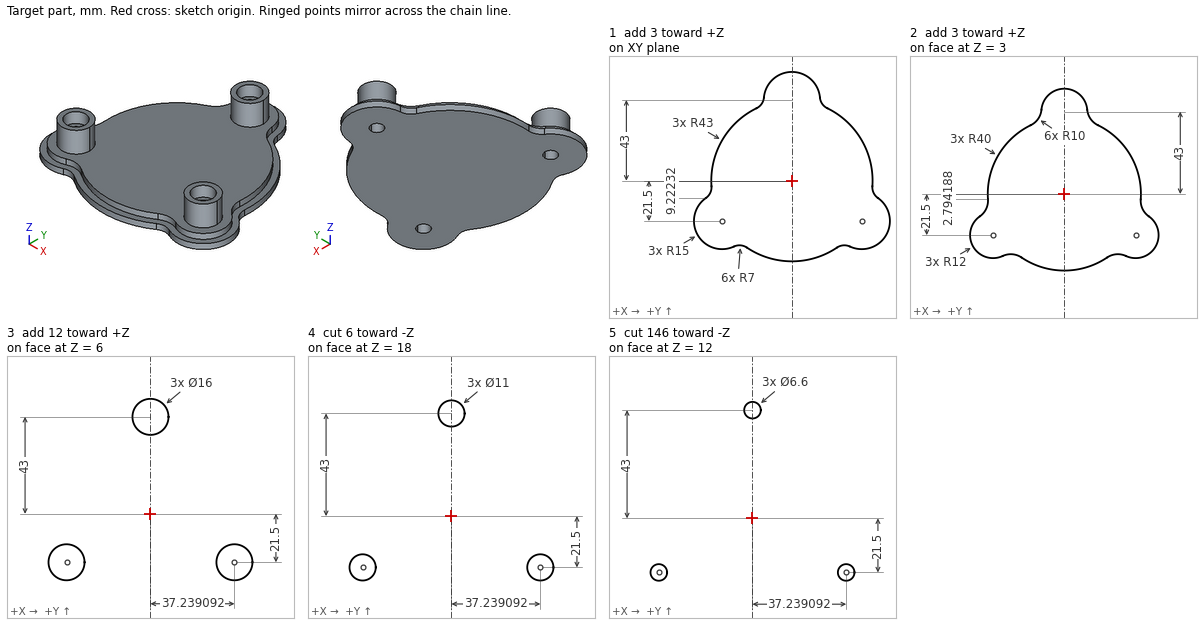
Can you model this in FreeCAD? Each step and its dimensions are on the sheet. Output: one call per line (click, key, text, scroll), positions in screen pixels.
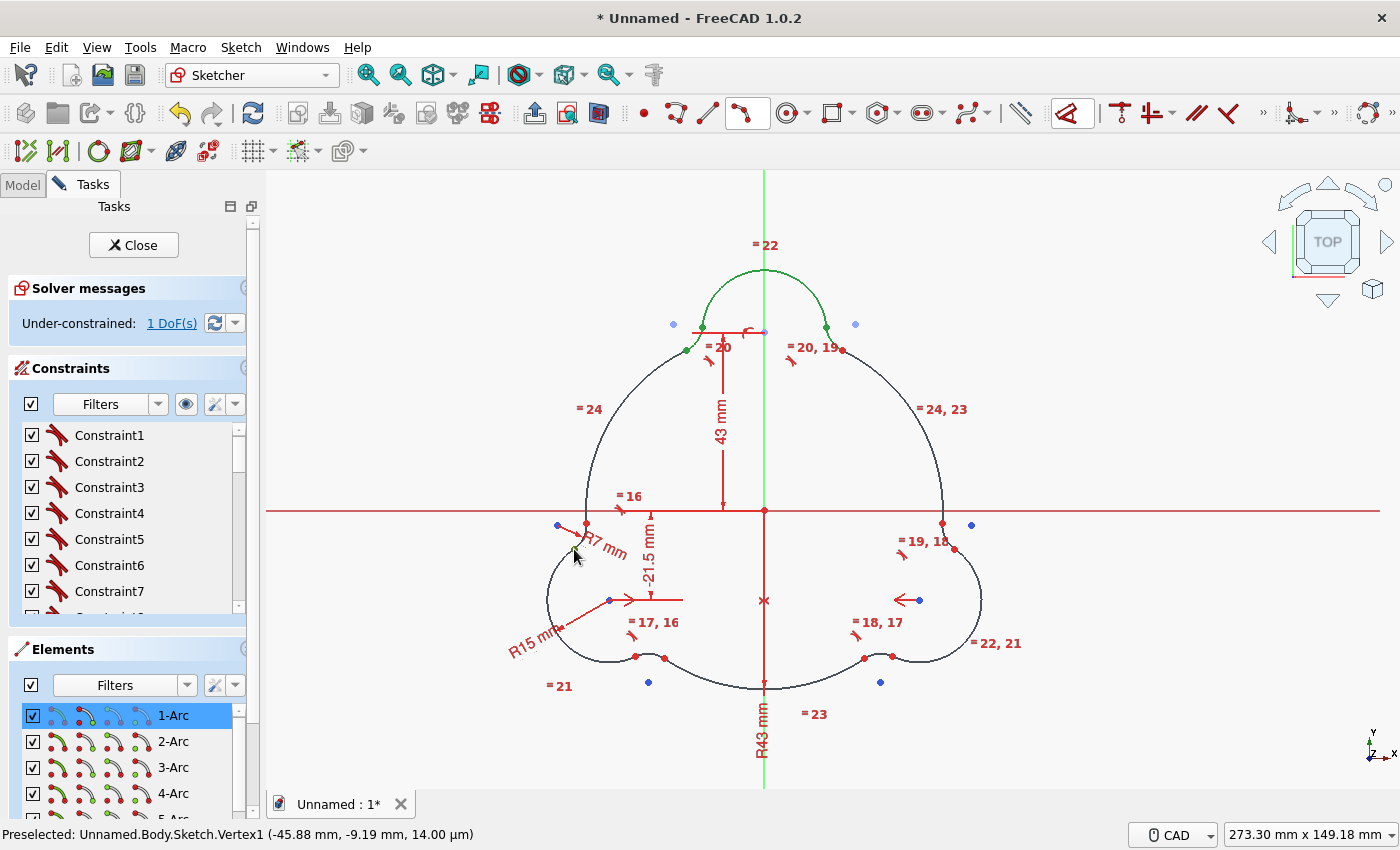
click(1088, 114)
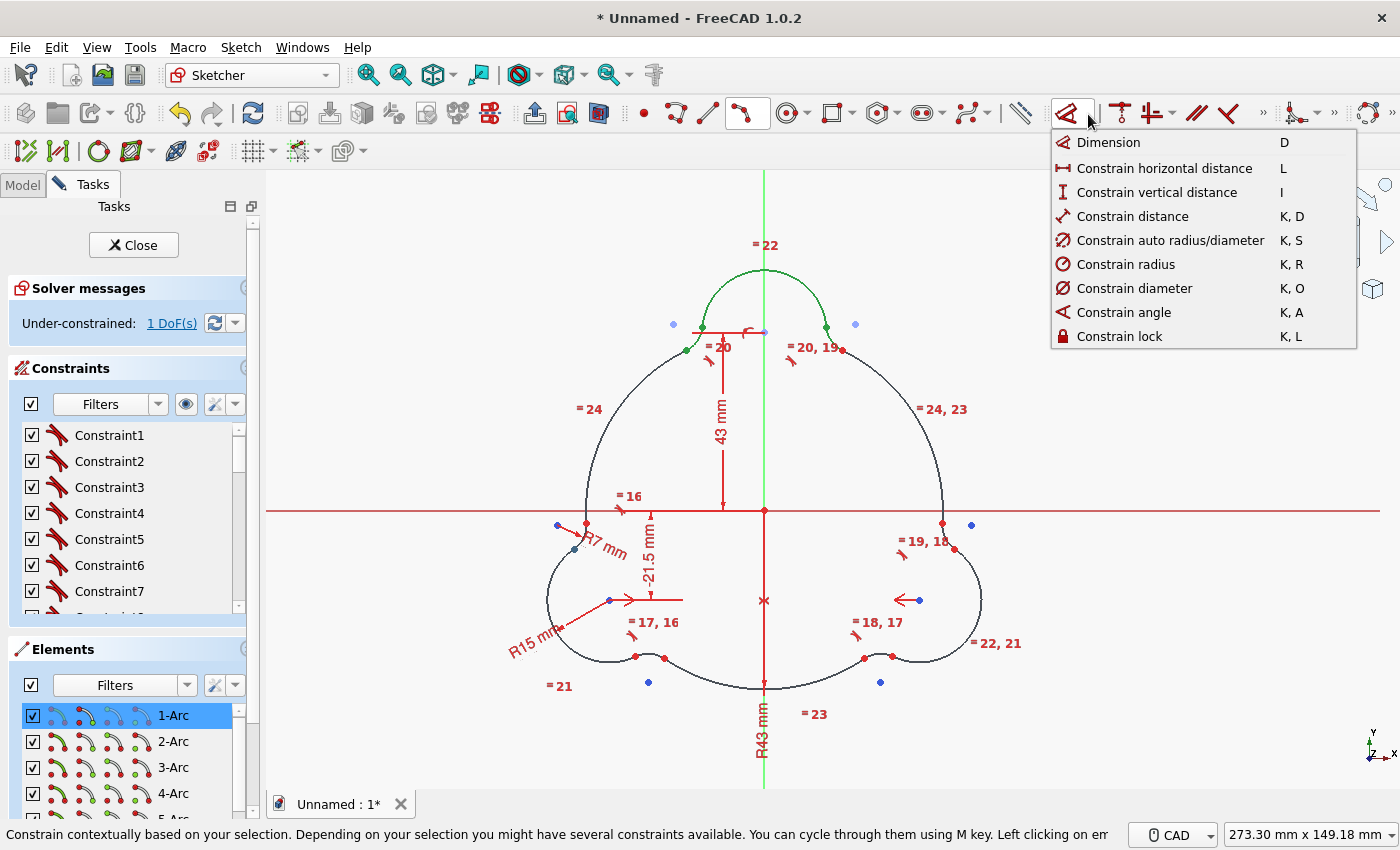
click(1204, 192)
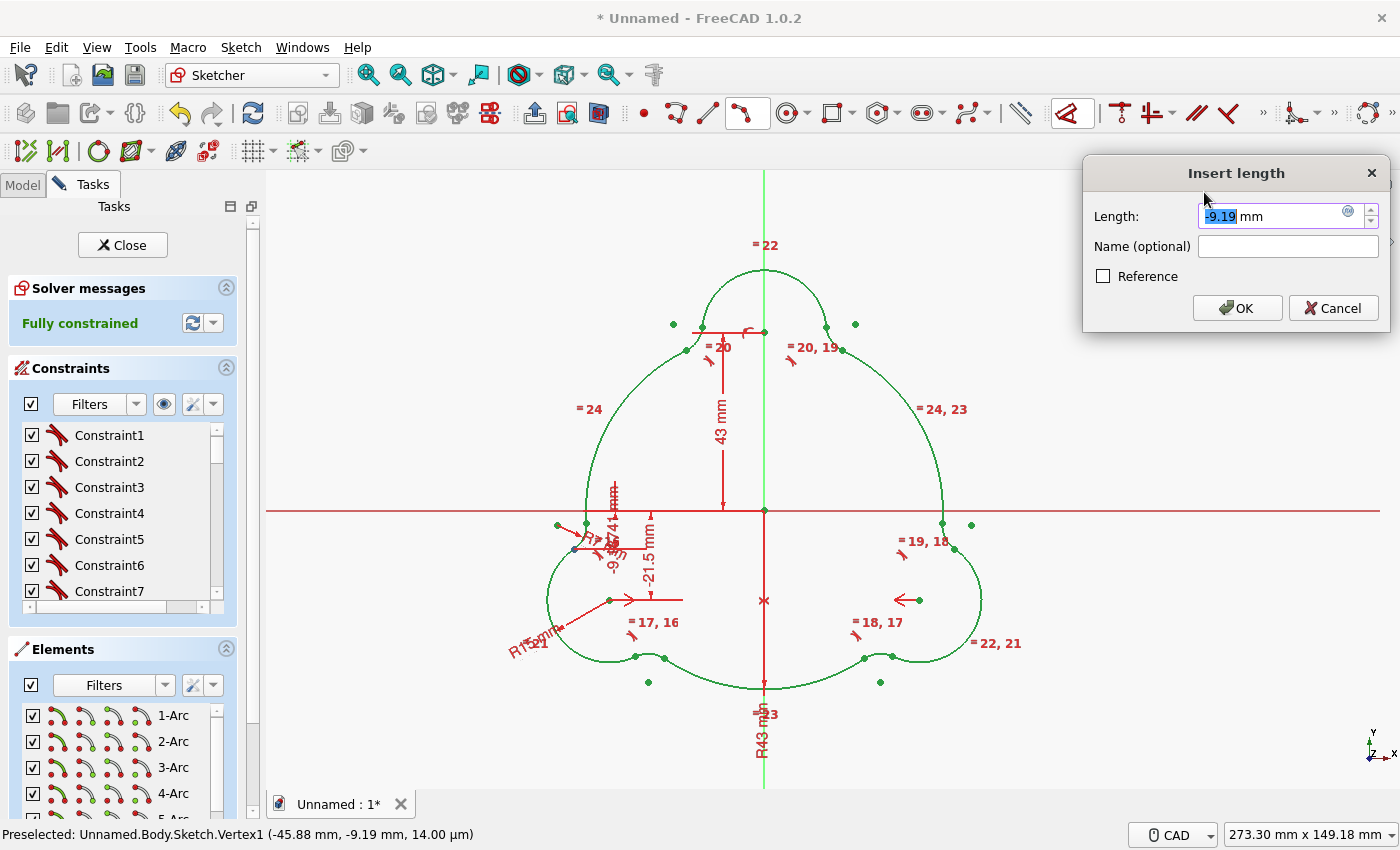
text(-9.22232)
key(Return)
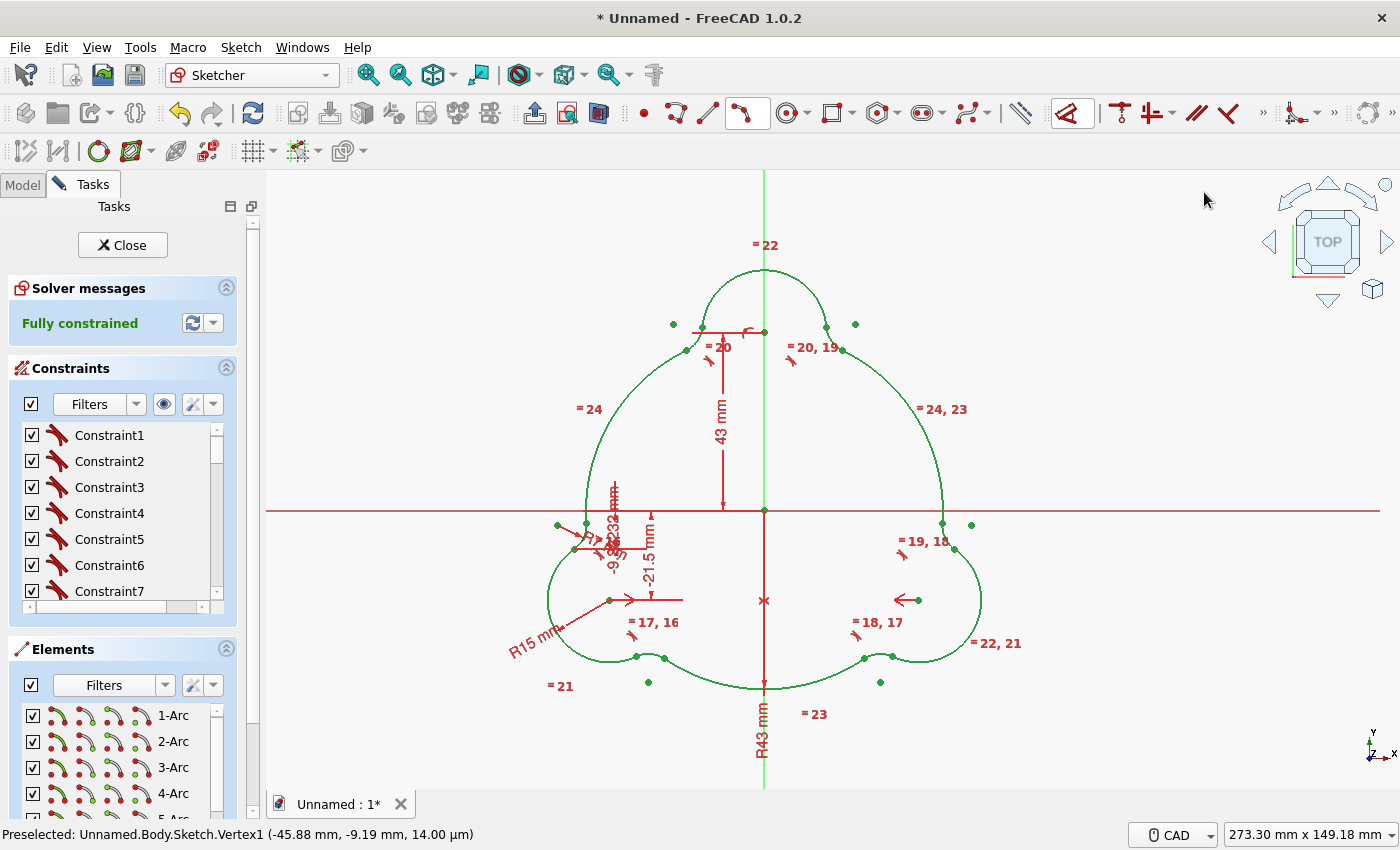
click(123, 245)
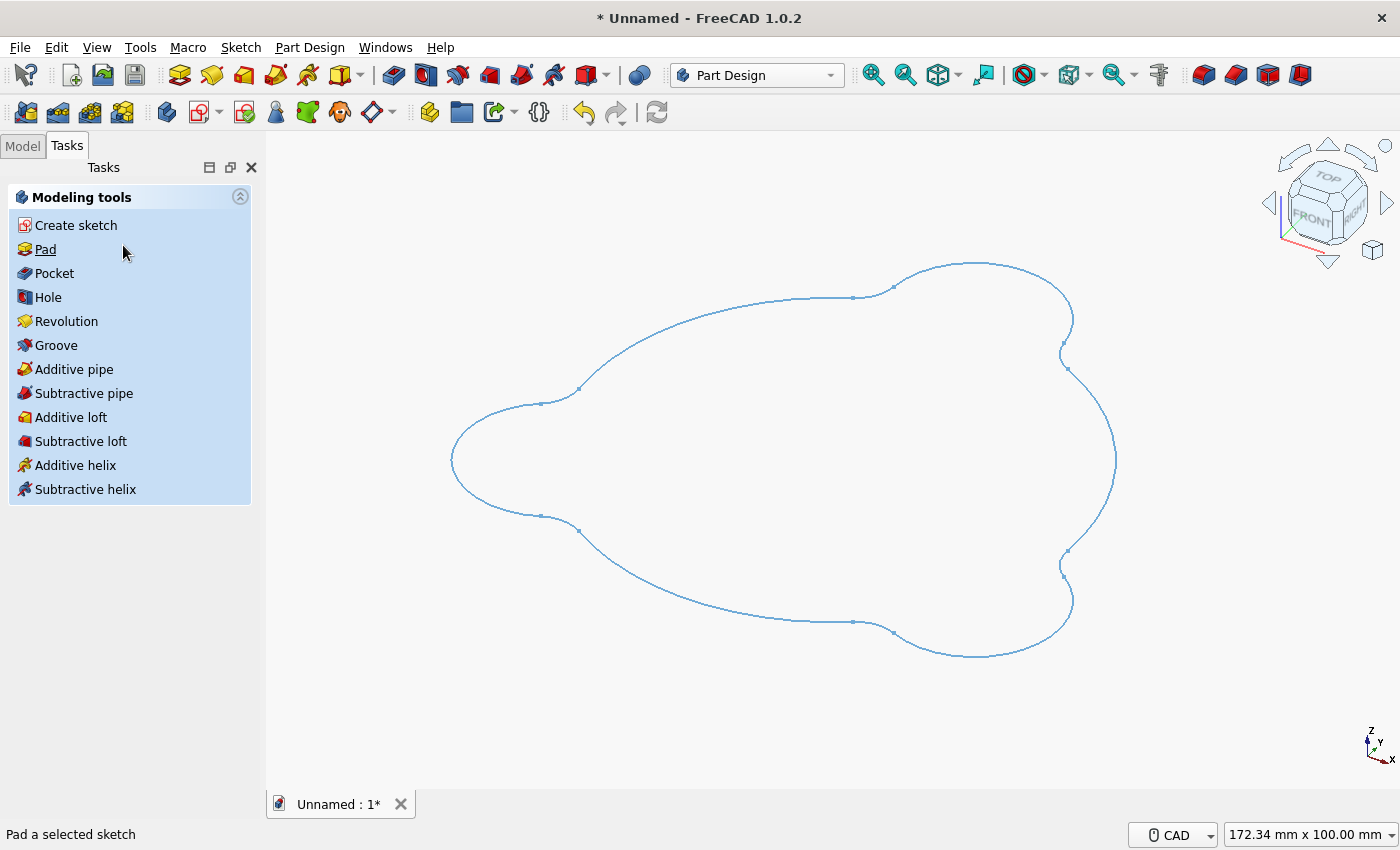
click(180, 76)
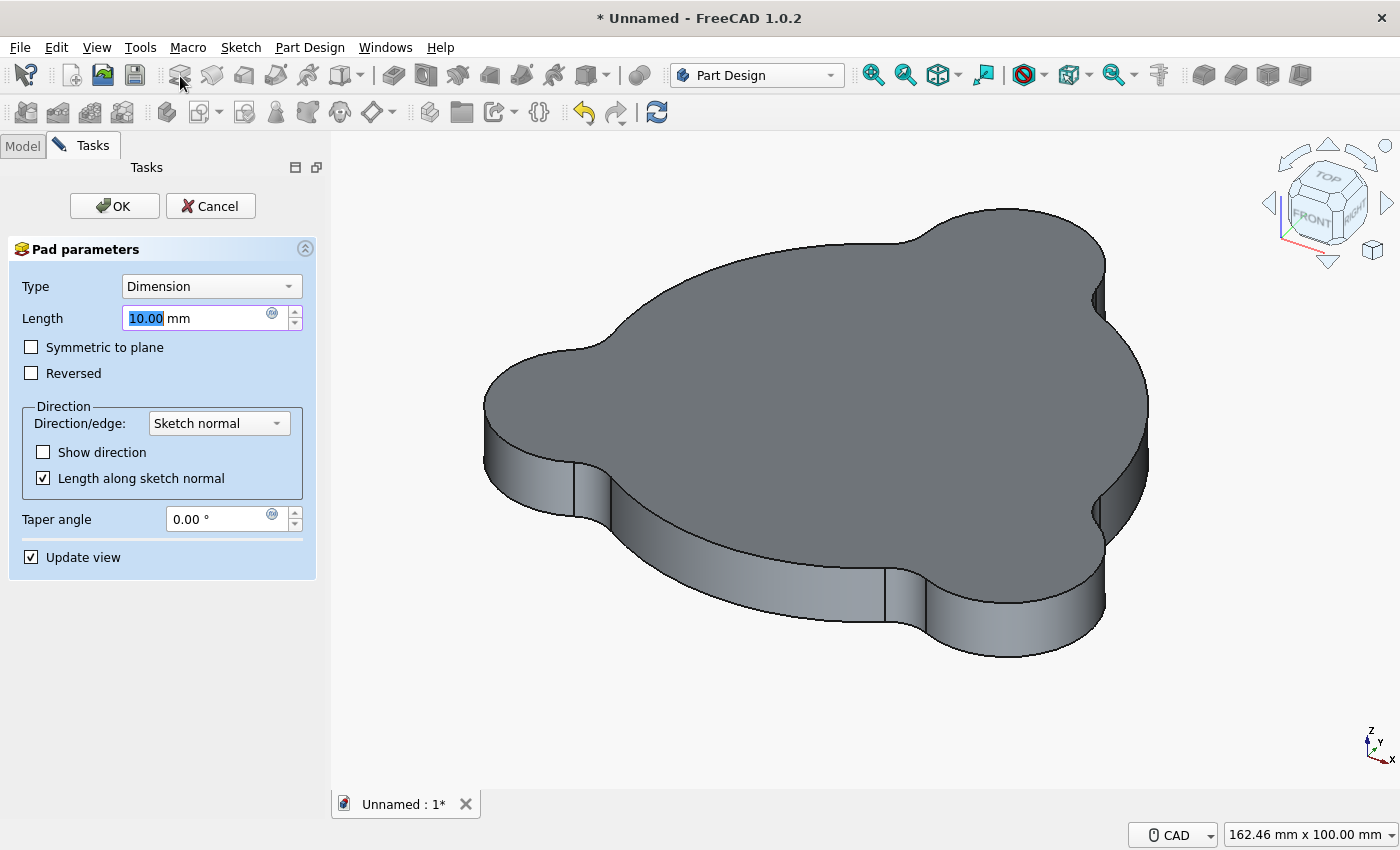
text(3)
key(Tab)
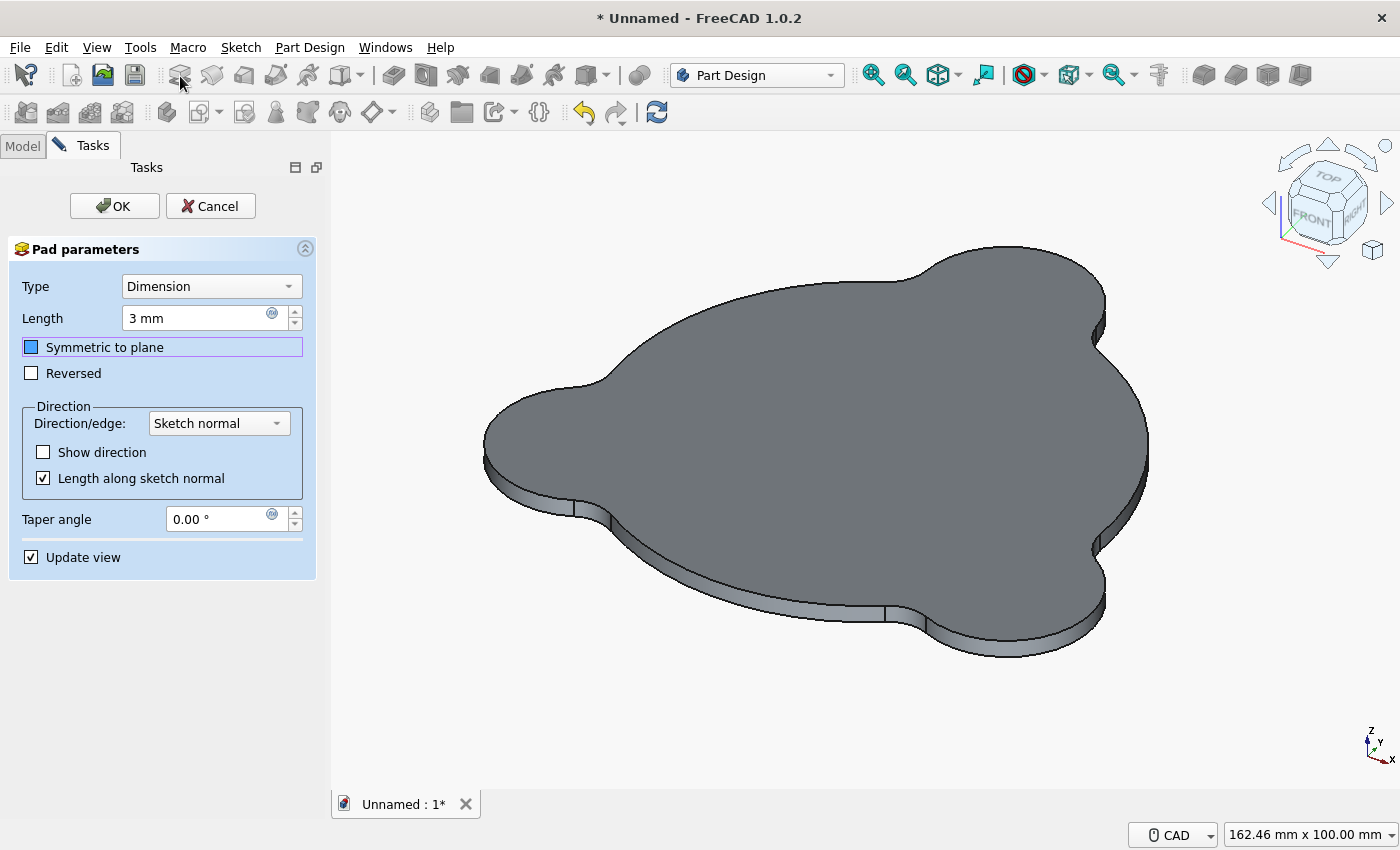
click(115, 206)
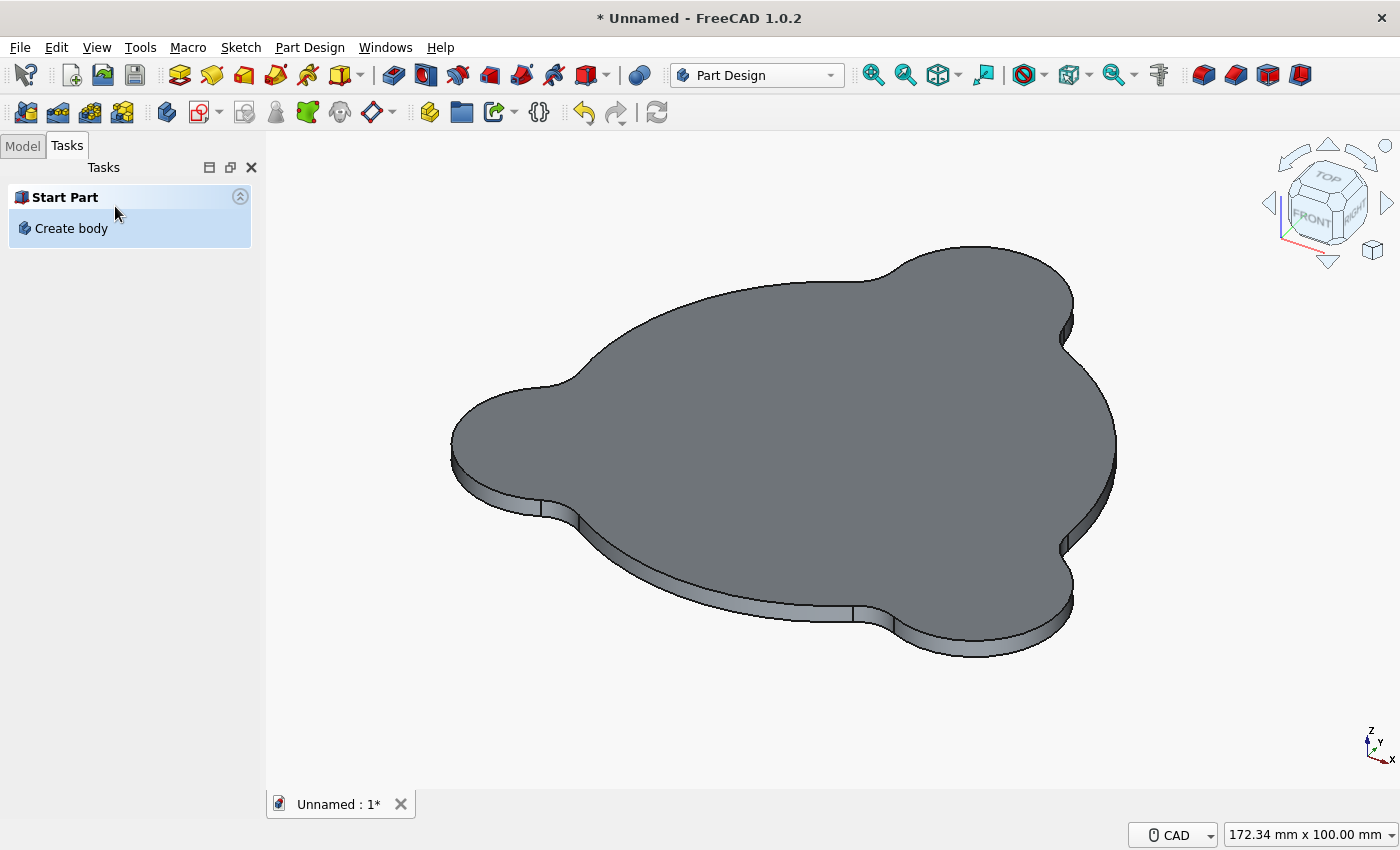
click(858, 418)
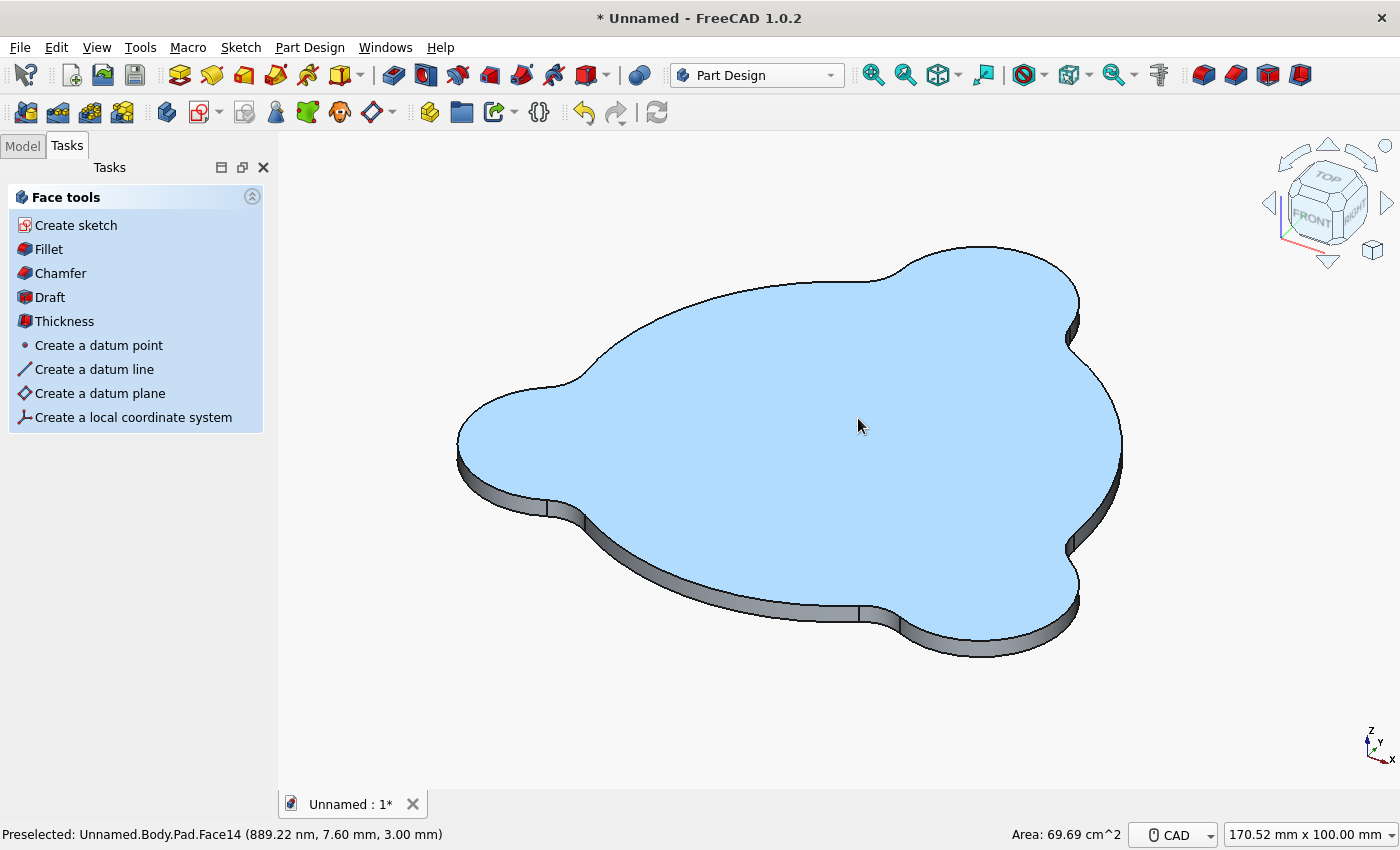
click(200, 112)